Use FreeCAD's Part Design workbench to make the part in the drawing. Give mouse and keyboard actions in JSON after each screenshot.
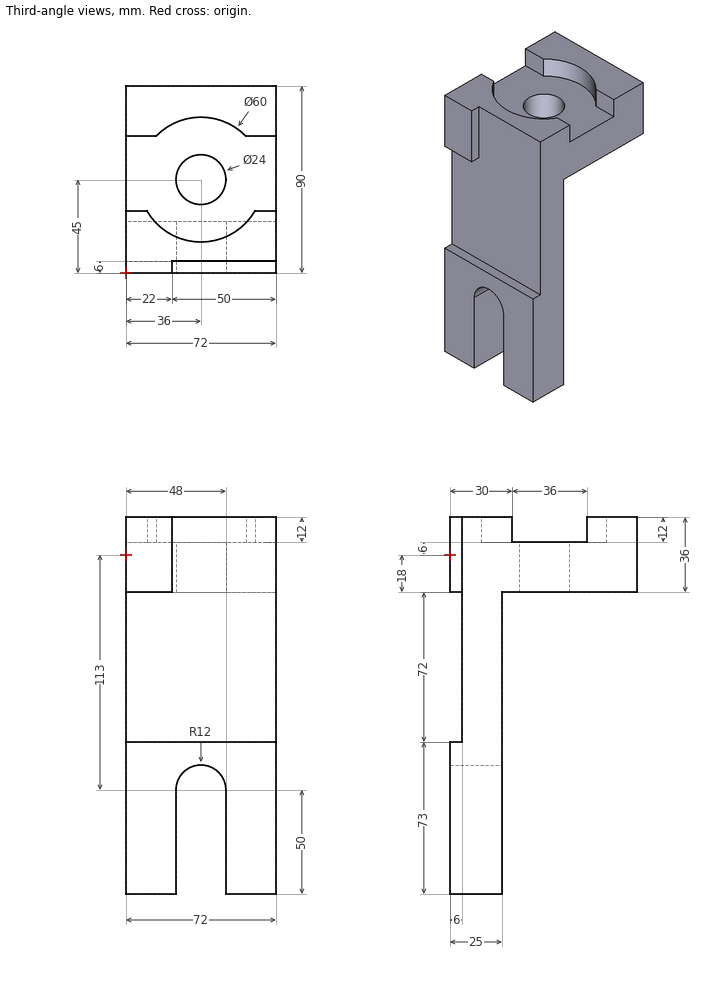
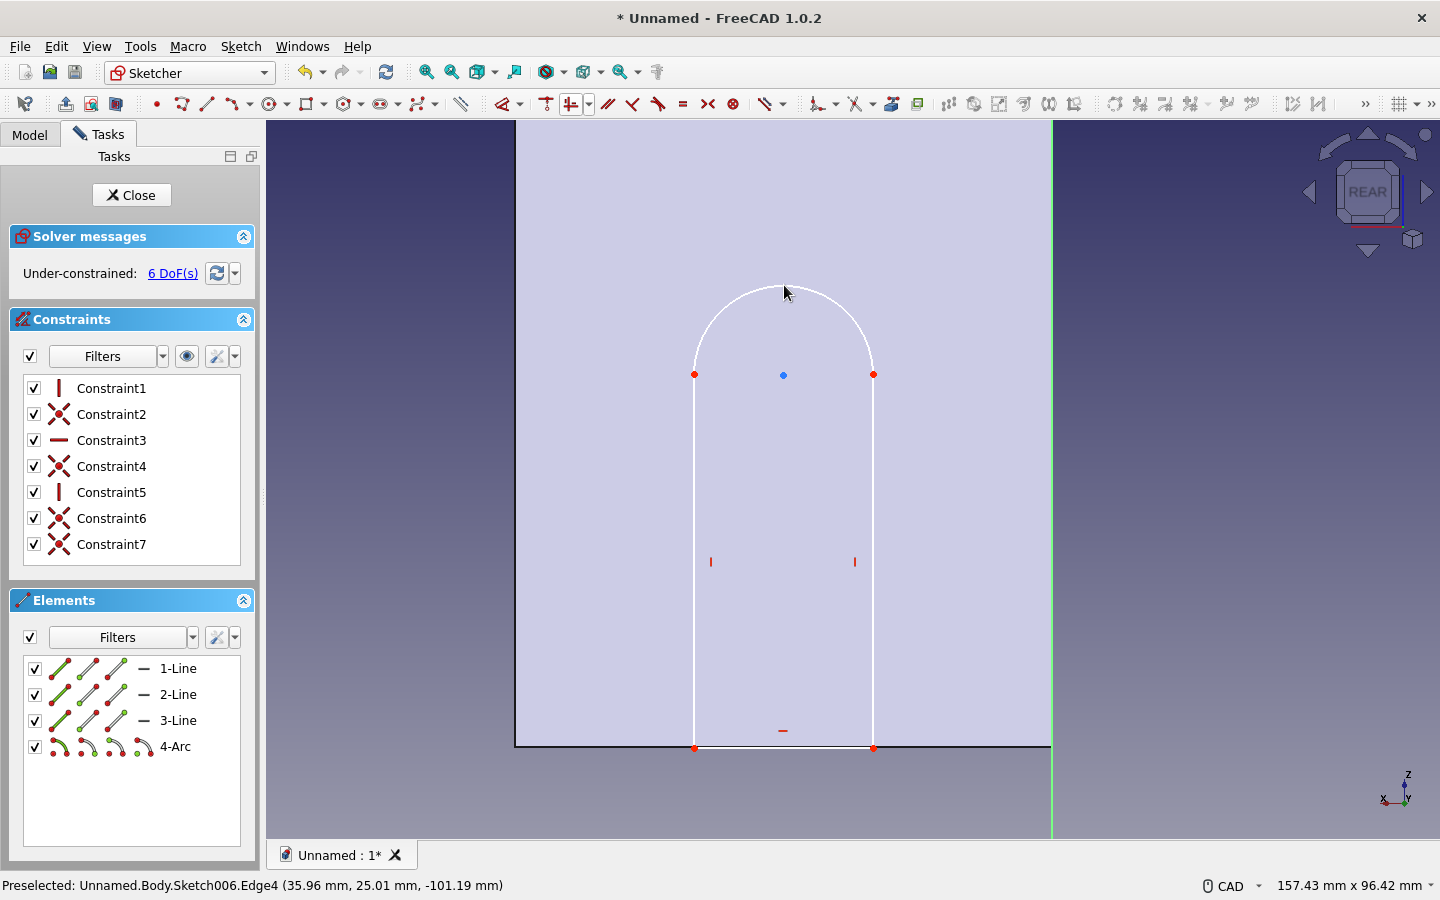
{"action": "left_click", "coordinate": [694, 487]}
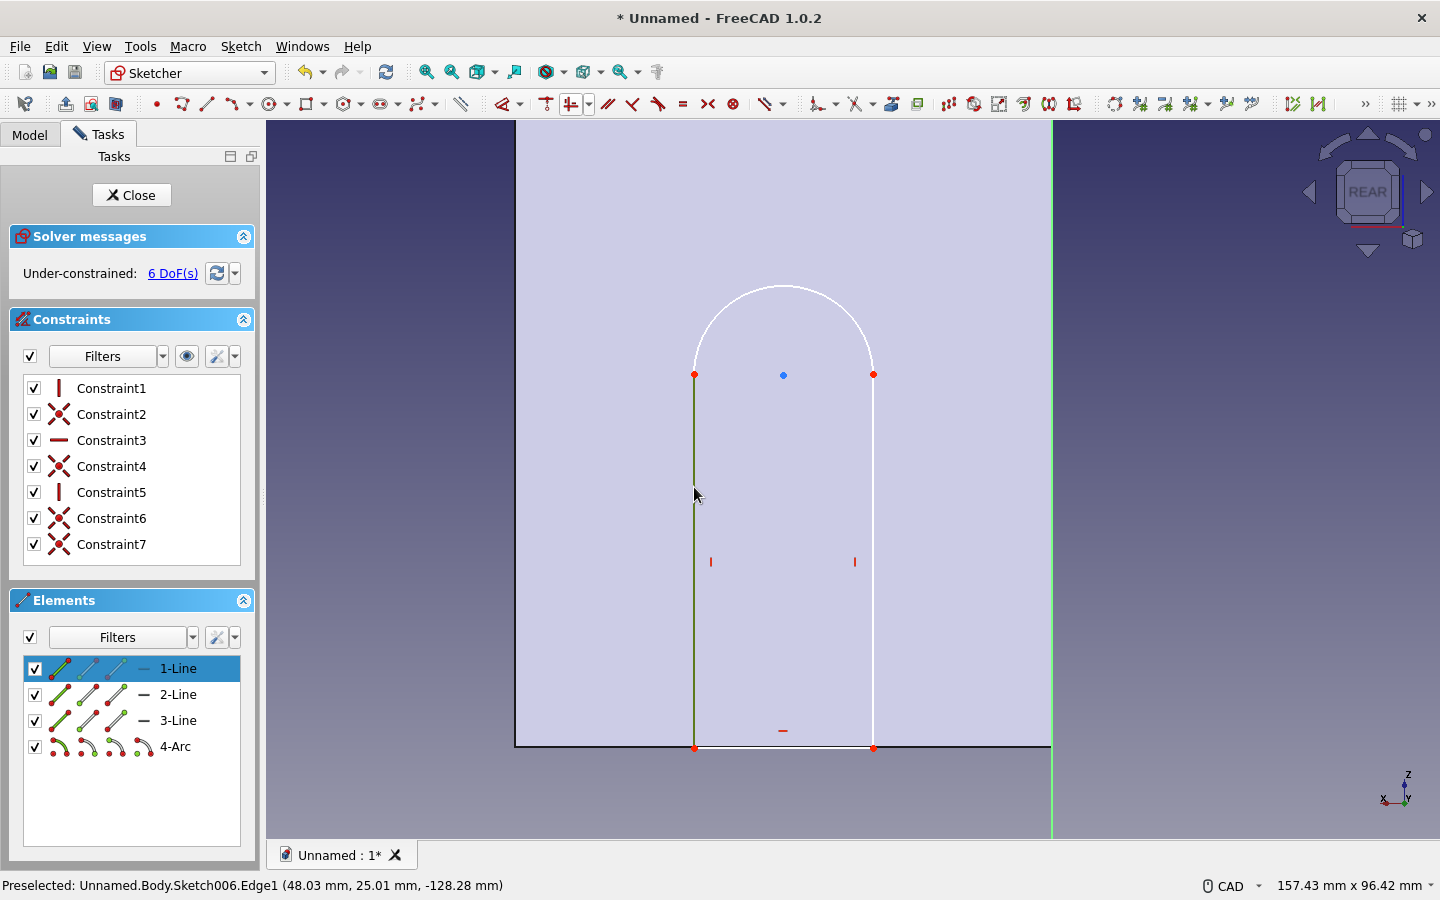
{"action": "left_click", "coordinate": [836, 303]}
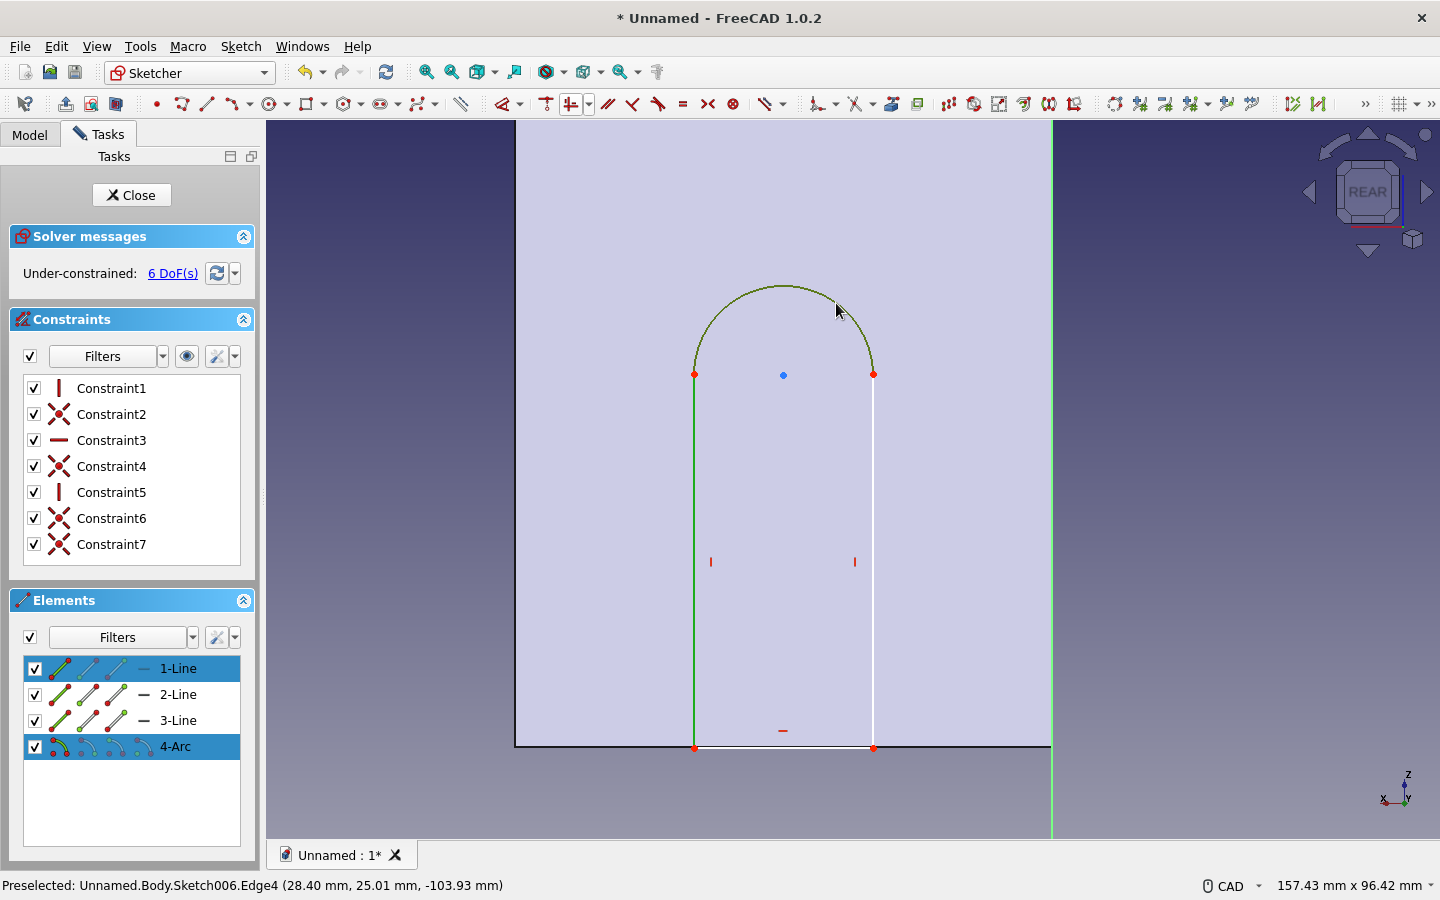
{"action": "key", "text": "t"}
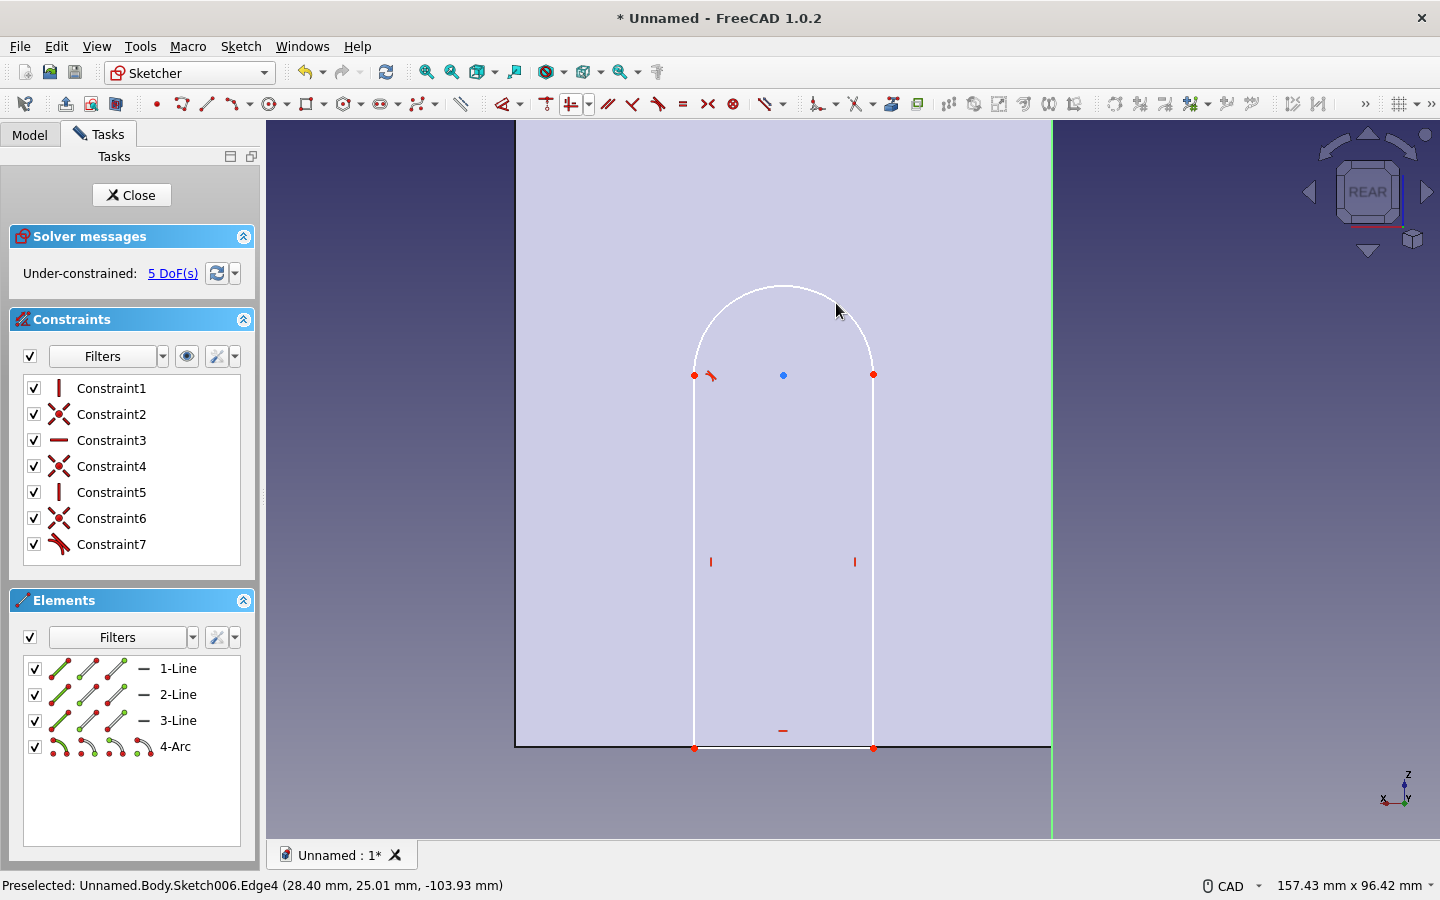
{"action": "left_click", "coordinate": [873, 636]}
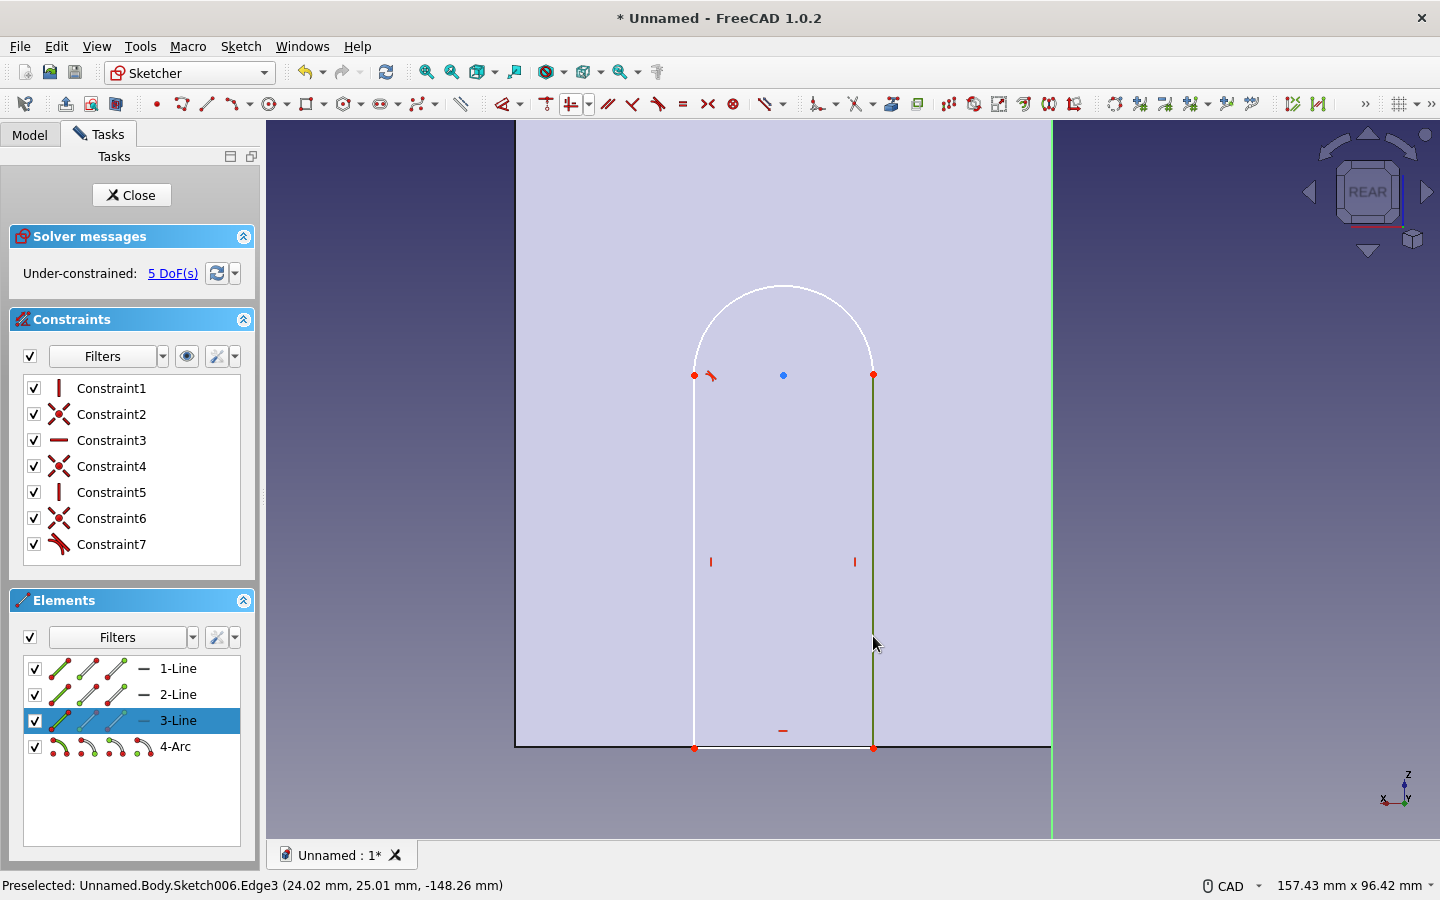
{"action": "left_click", "coordinate": [836, 303]}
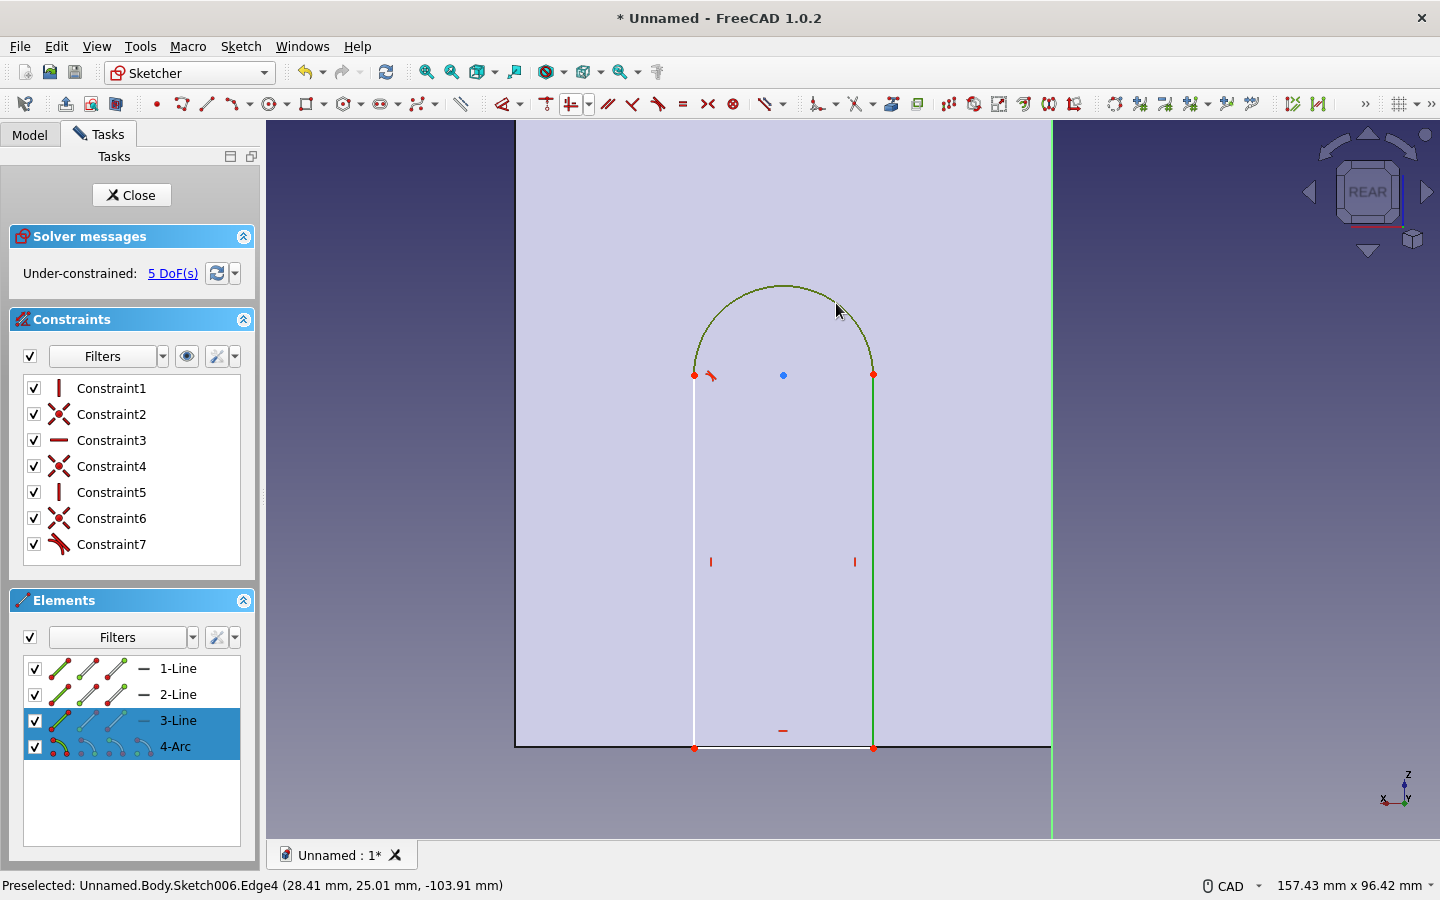
{"action": "key", "text": "t"}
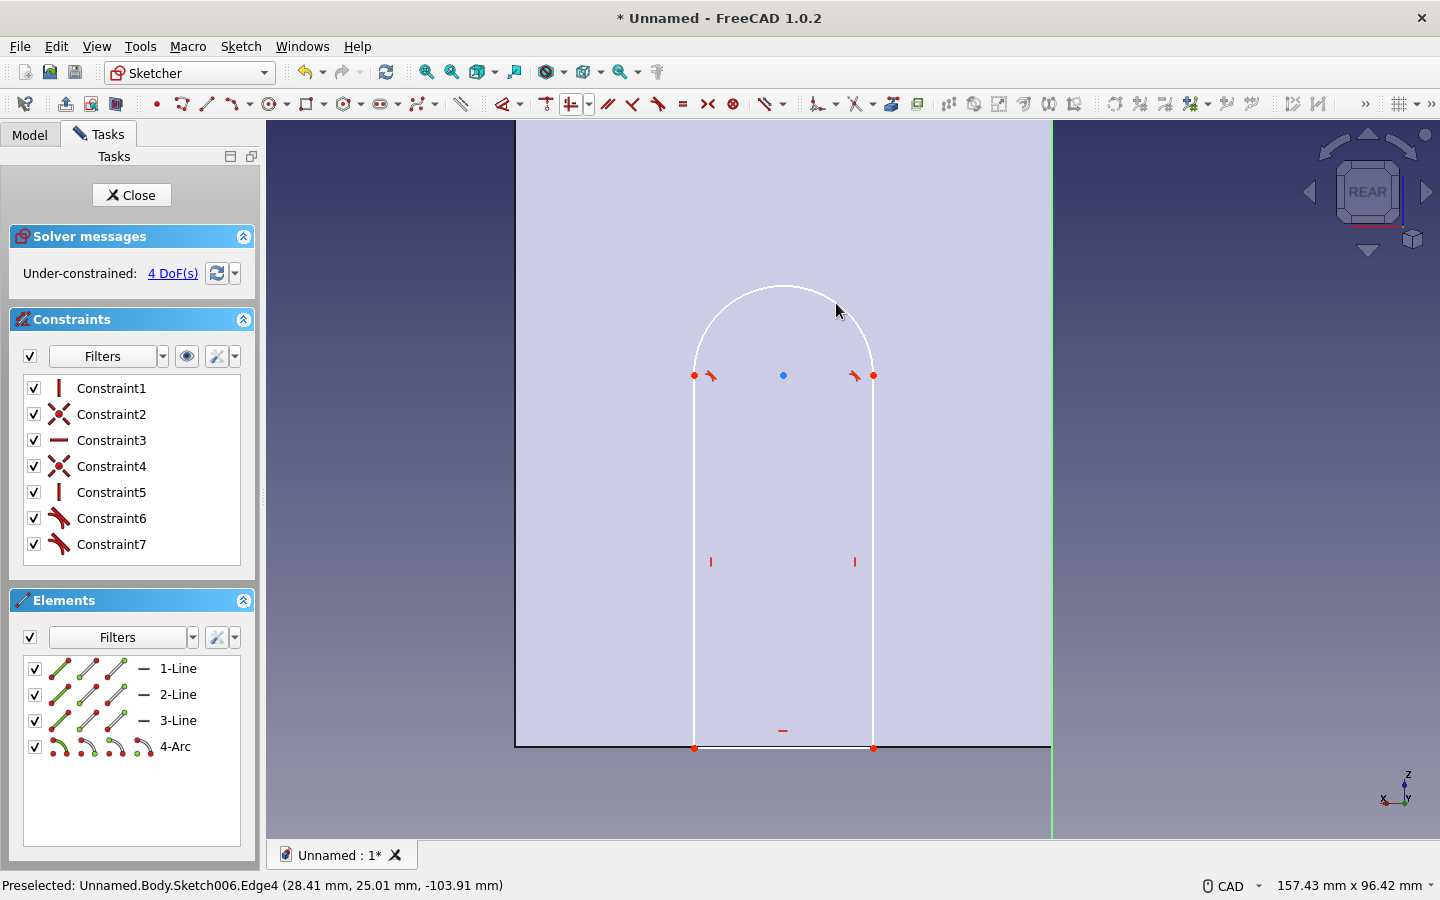
{"action": "key", "text": "d"}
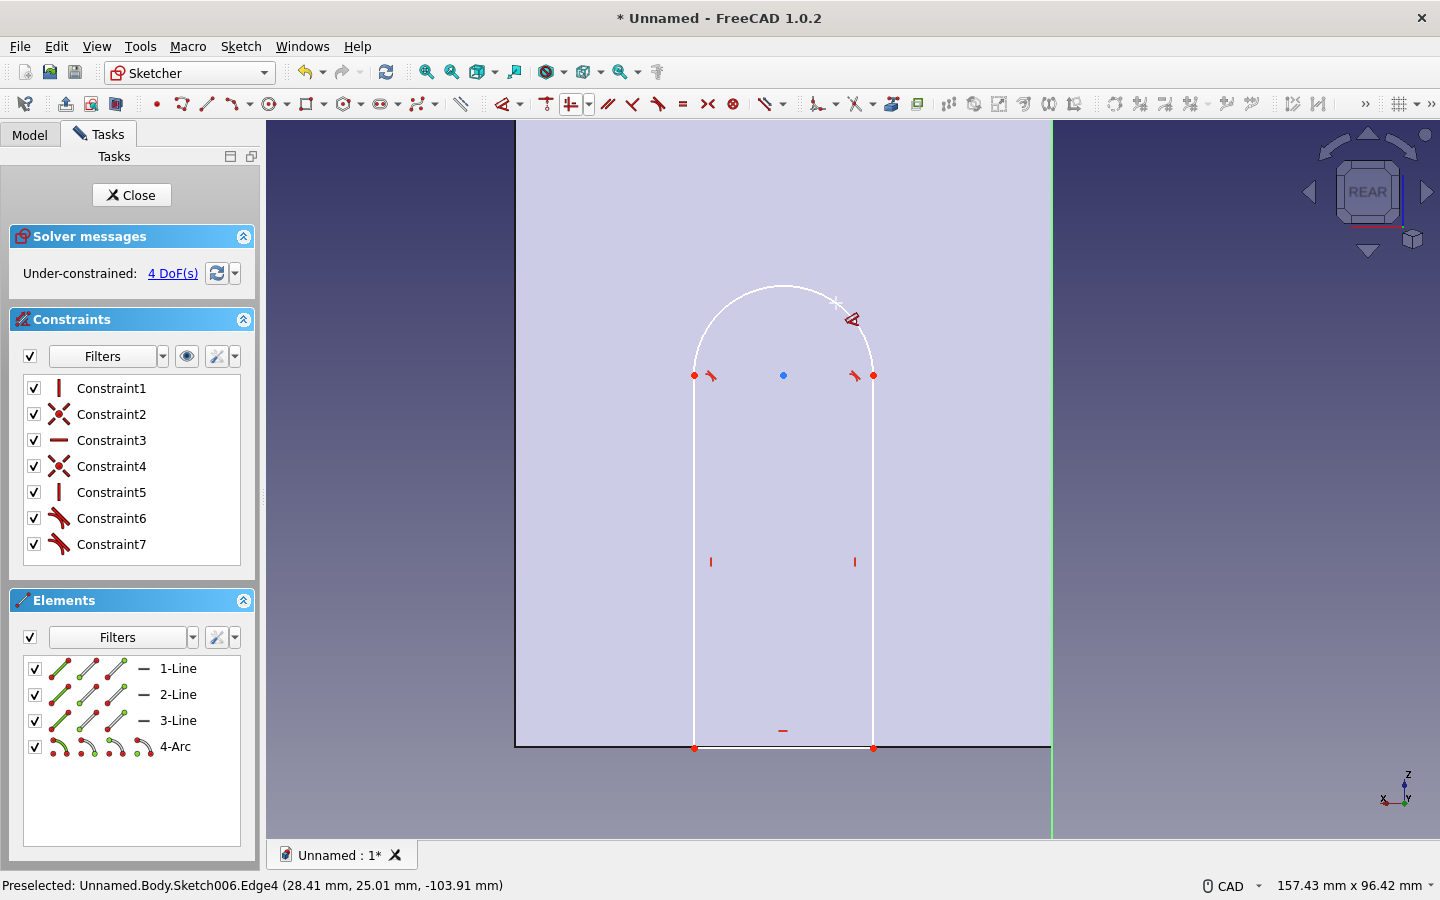
{"action": "left_click", "coordinate": [836, 303]}
{"action": "left_click", "coordinate": [855, 277]}